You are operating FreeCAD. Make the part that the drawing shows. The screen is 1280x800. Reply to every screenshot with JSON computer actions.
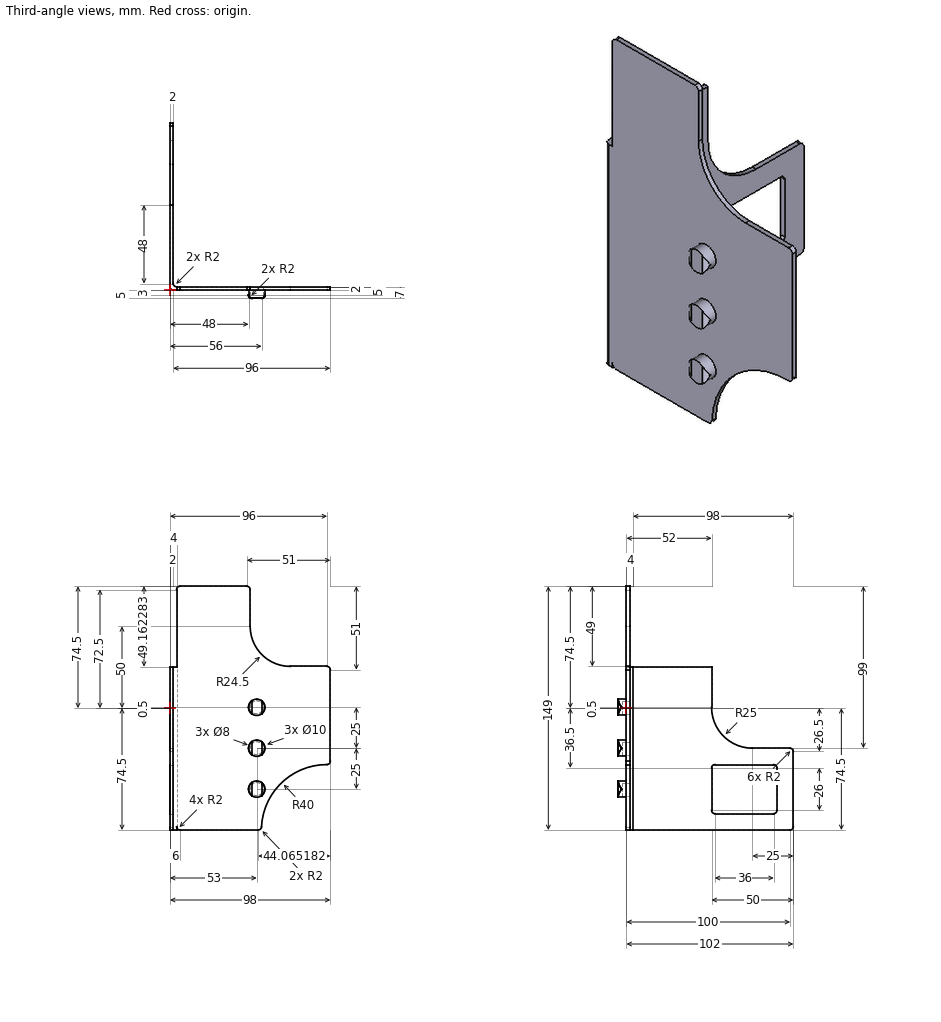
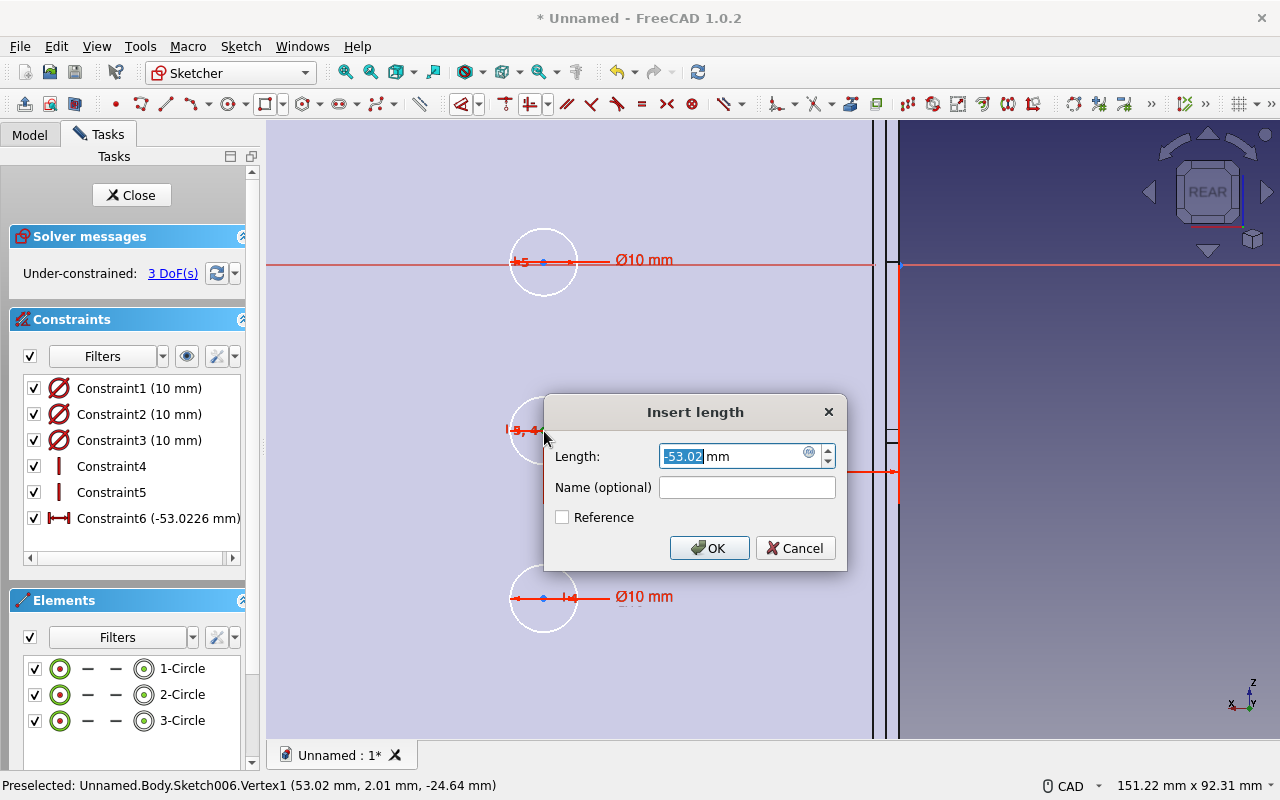
{"action": "type", "text": "-53"}
{"action": "key", "text": "Return"}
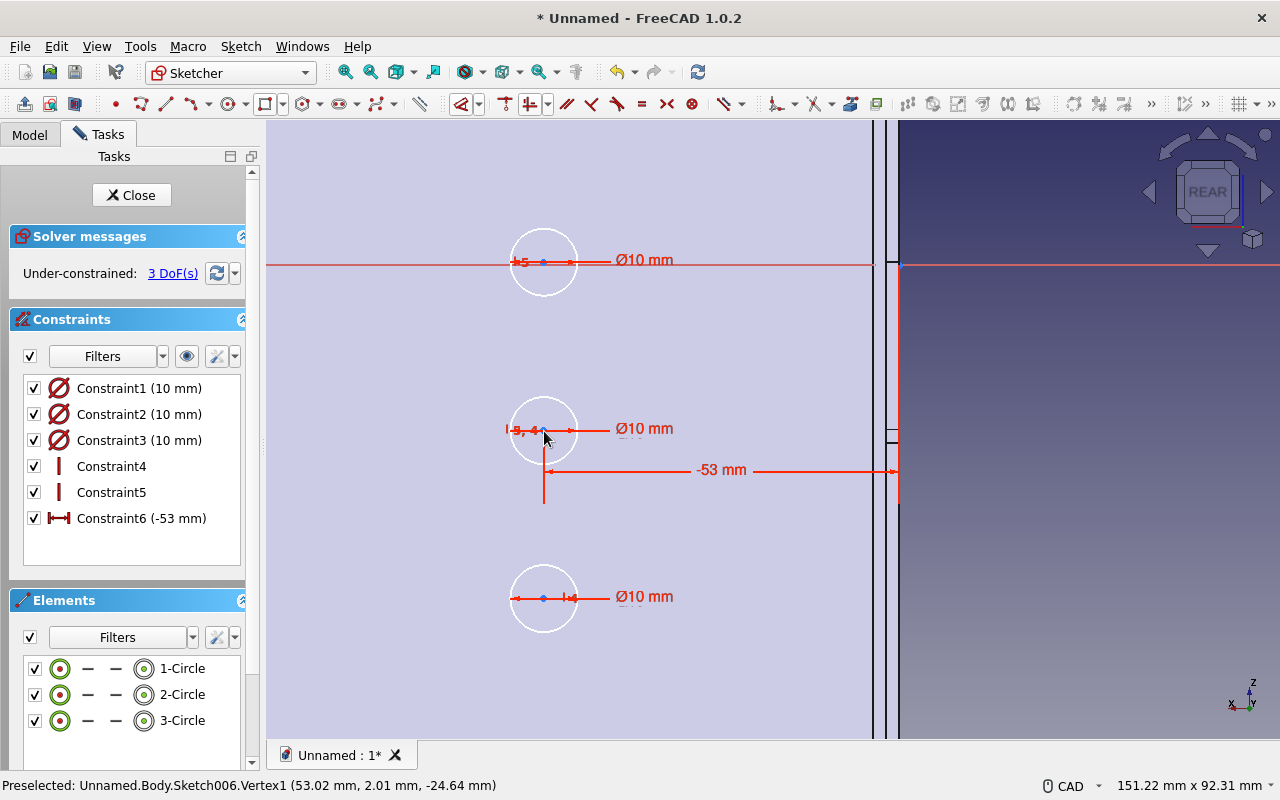
{"action": "scroll", "coordinate": [544, 262], "scroll_direction": "up", "scroll_amount": 13}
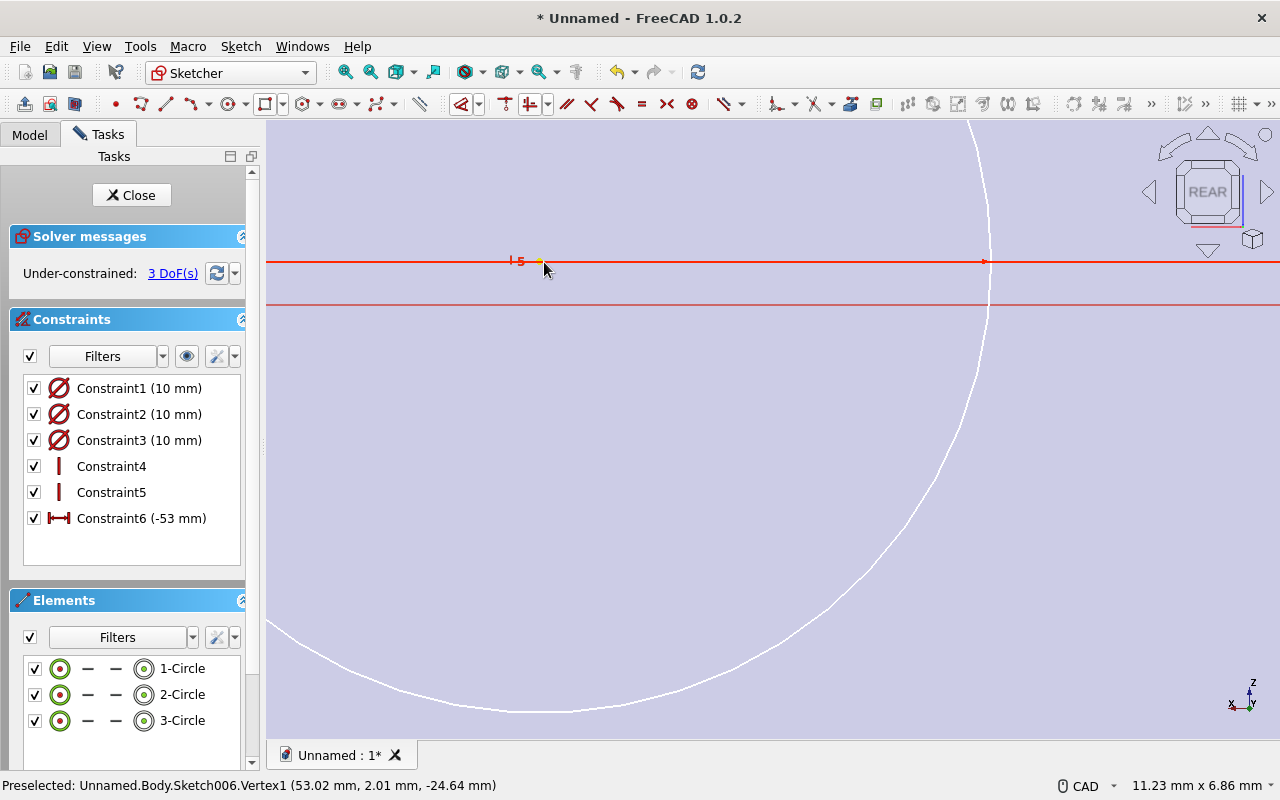
{"action": "left_click", "coordinate": [540, 262]}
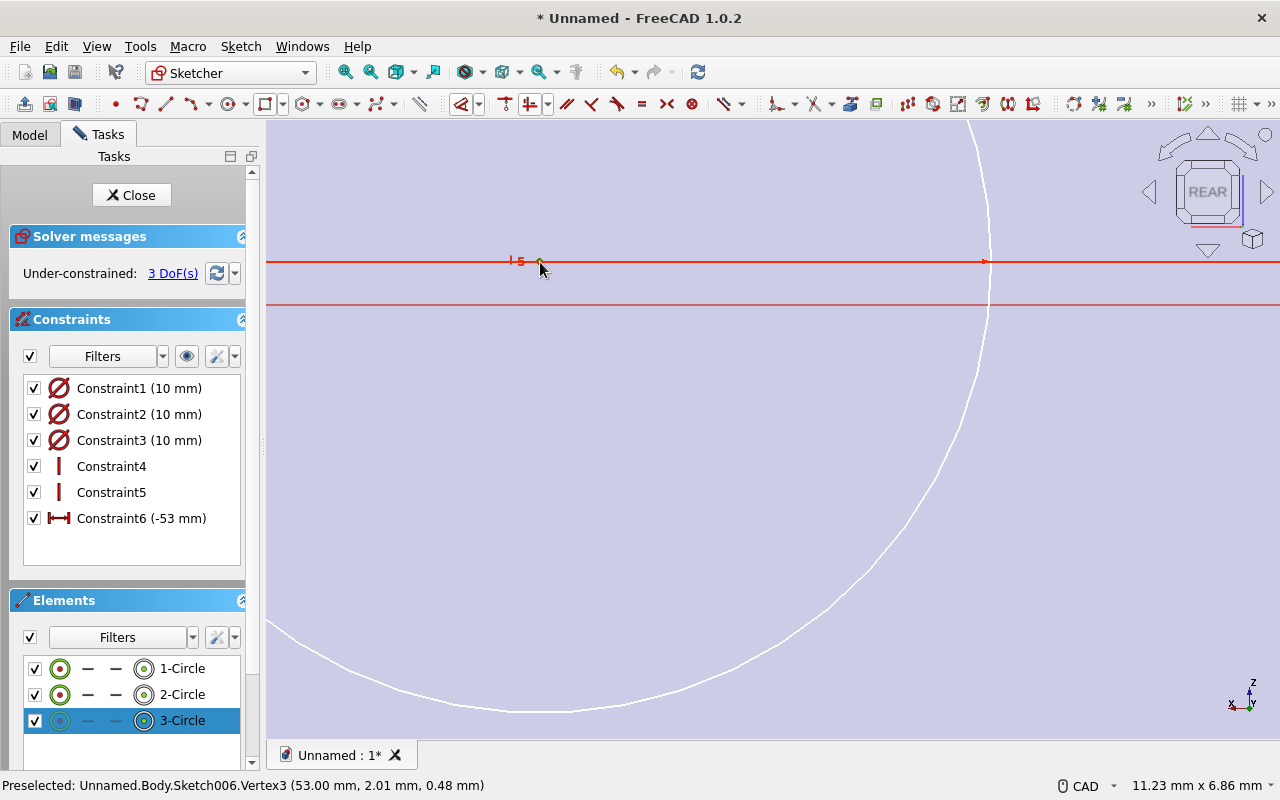
{"action": "key", "text": "i"}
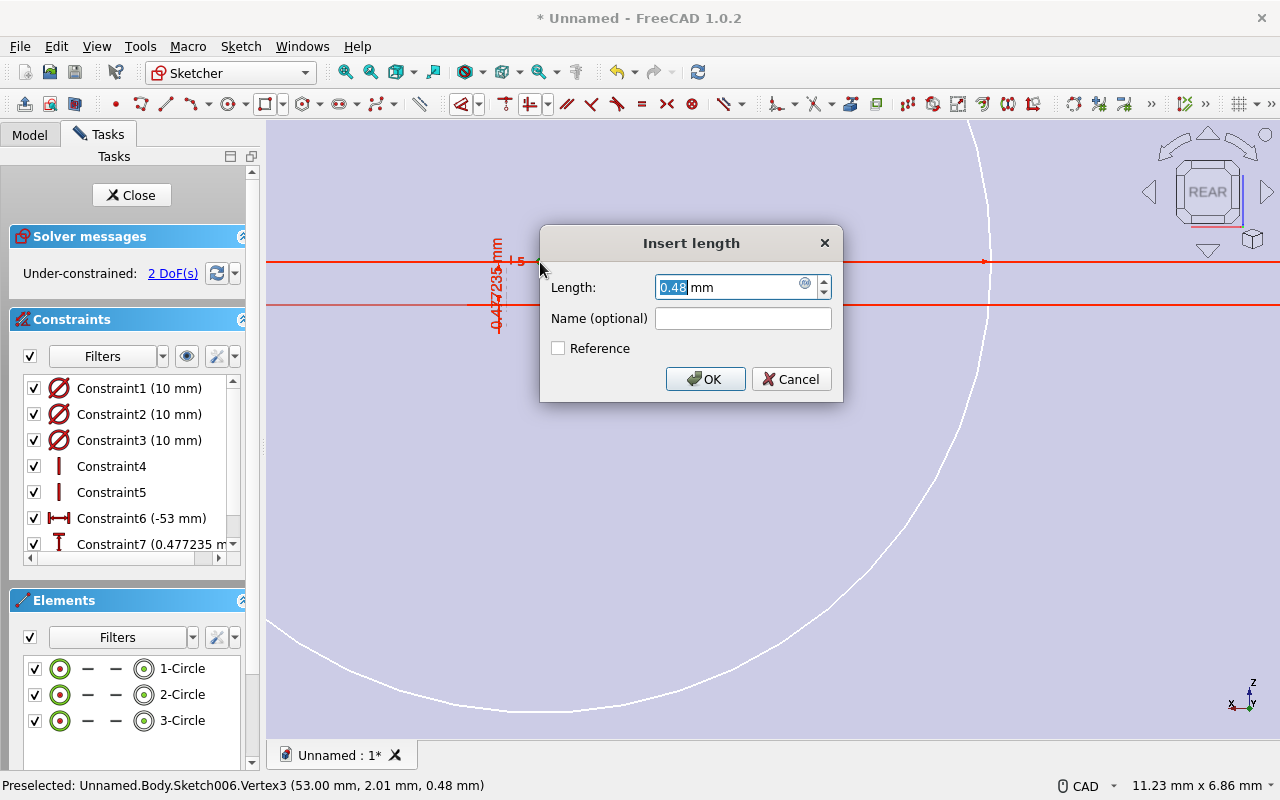
{"action": "type", "text": "0.5"}
{"action": "key", "text": "Return"}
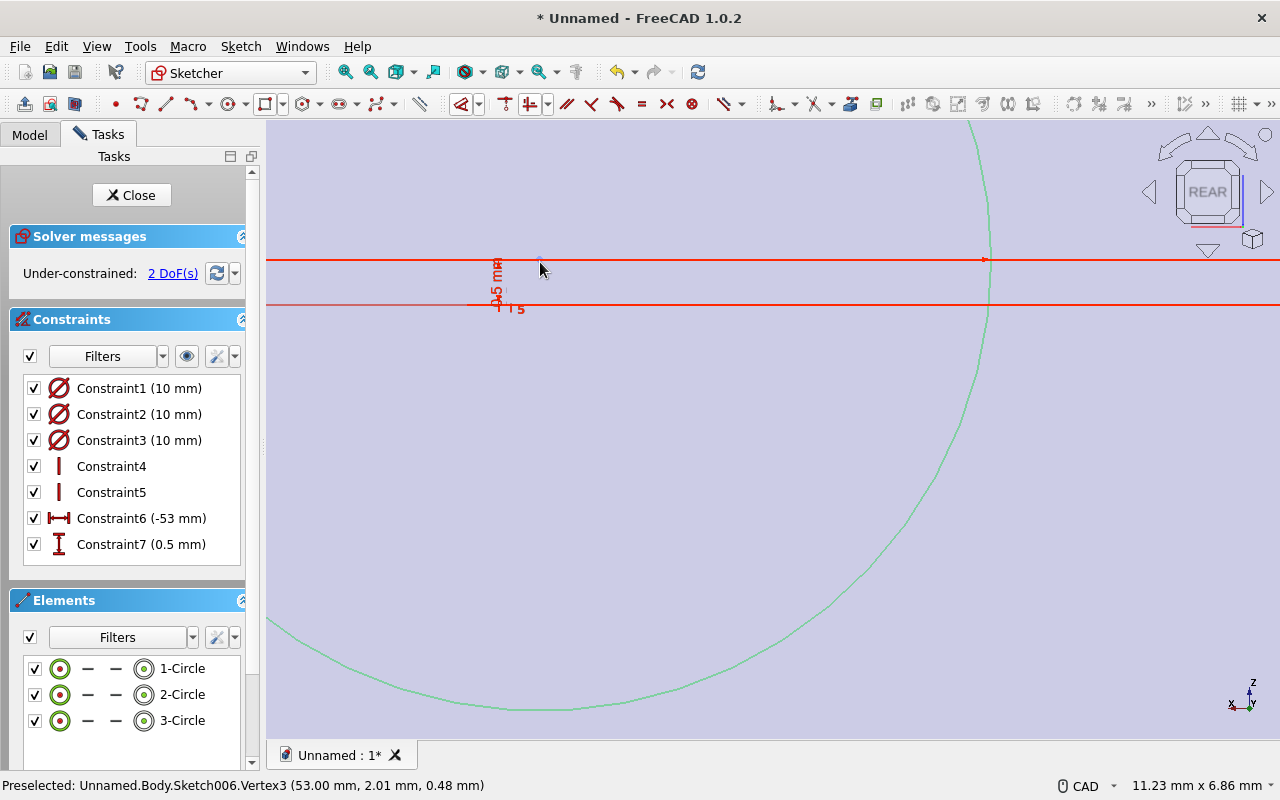
{"action": "scroll", "coordinate": [544, 262], "scroll_direction": "down", "scroll_amount": 13}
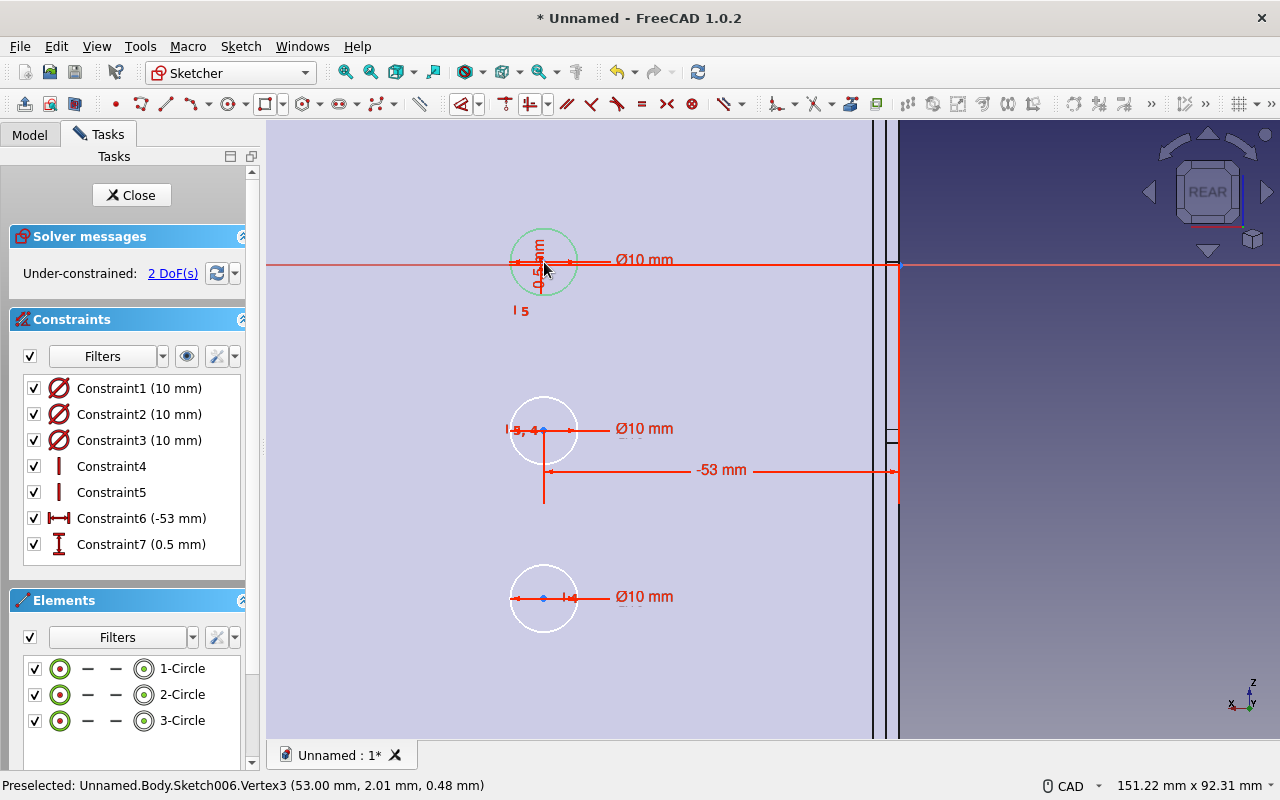
{"action": "left_click", "coordinate": [544, 431]}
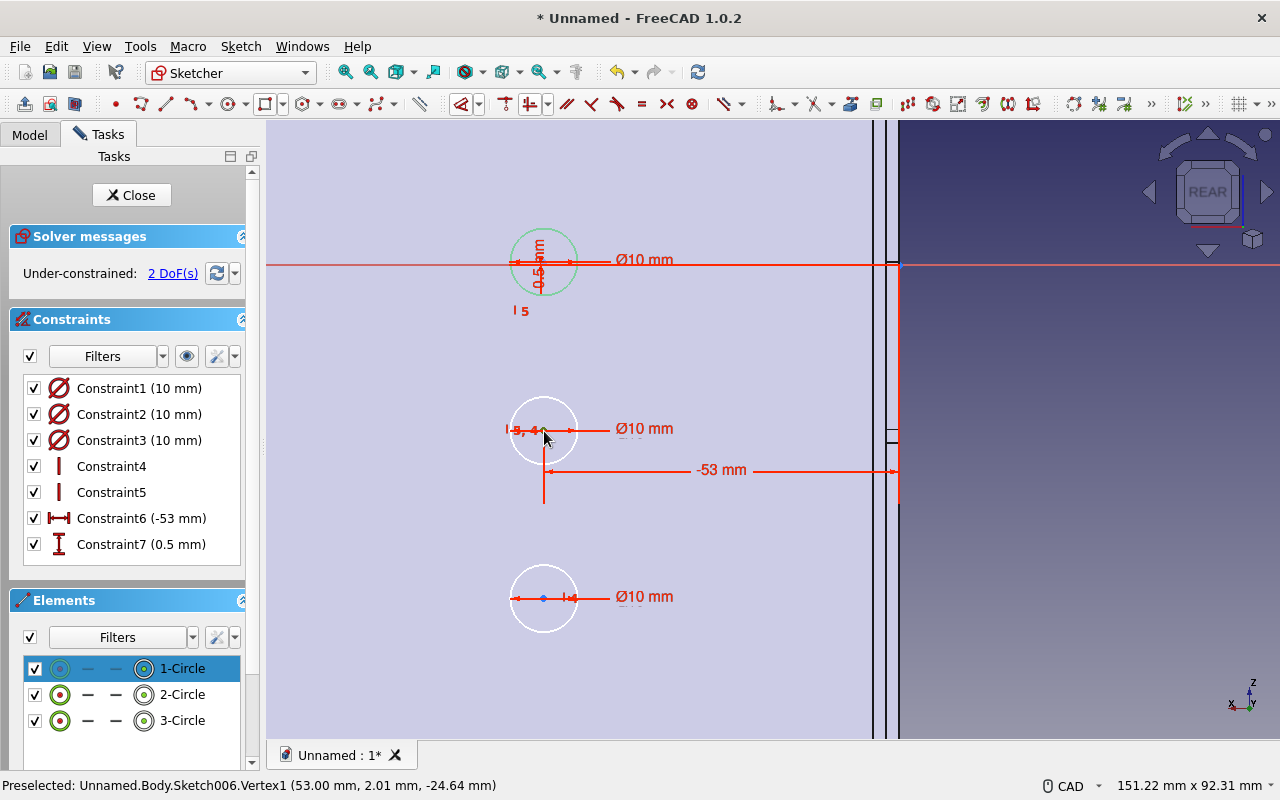
{"action": "left_click", "coordinate": [544, 599]}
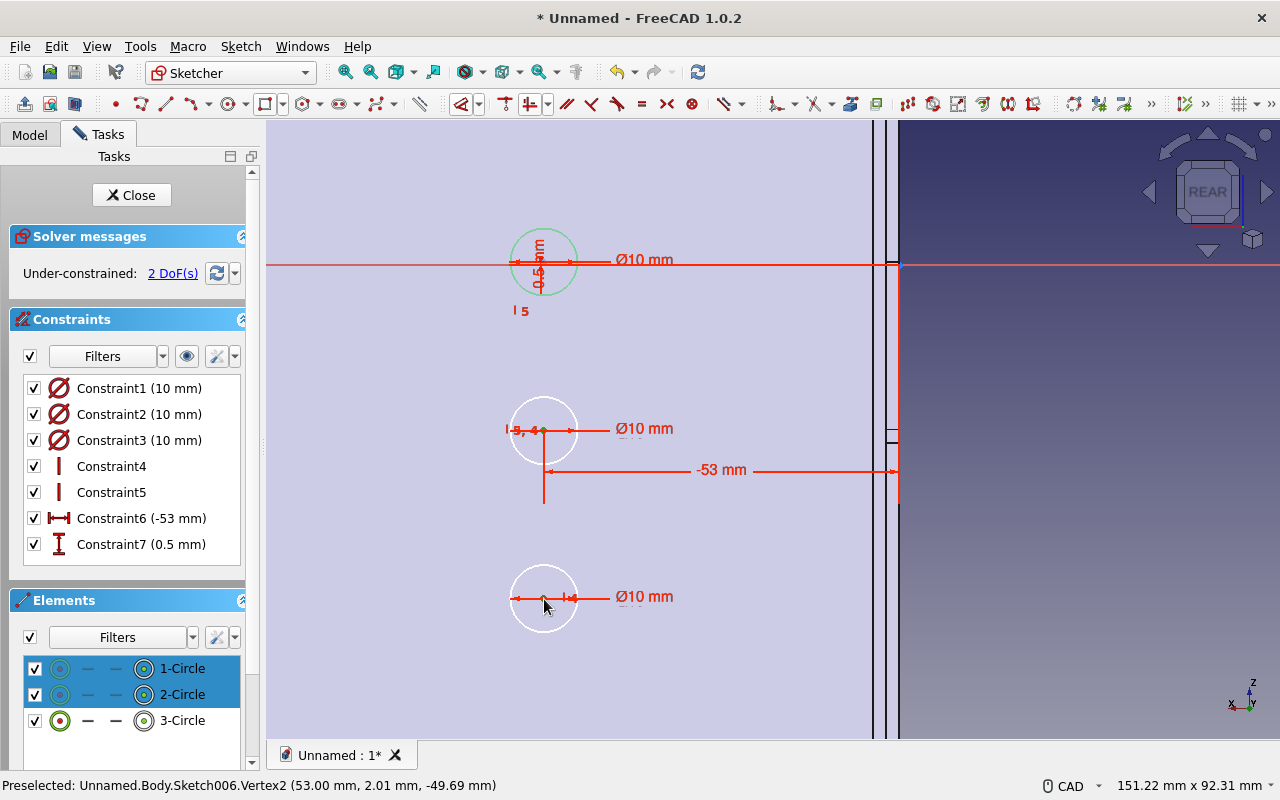
{"action": "left_click", "coordinate": [478, 104]}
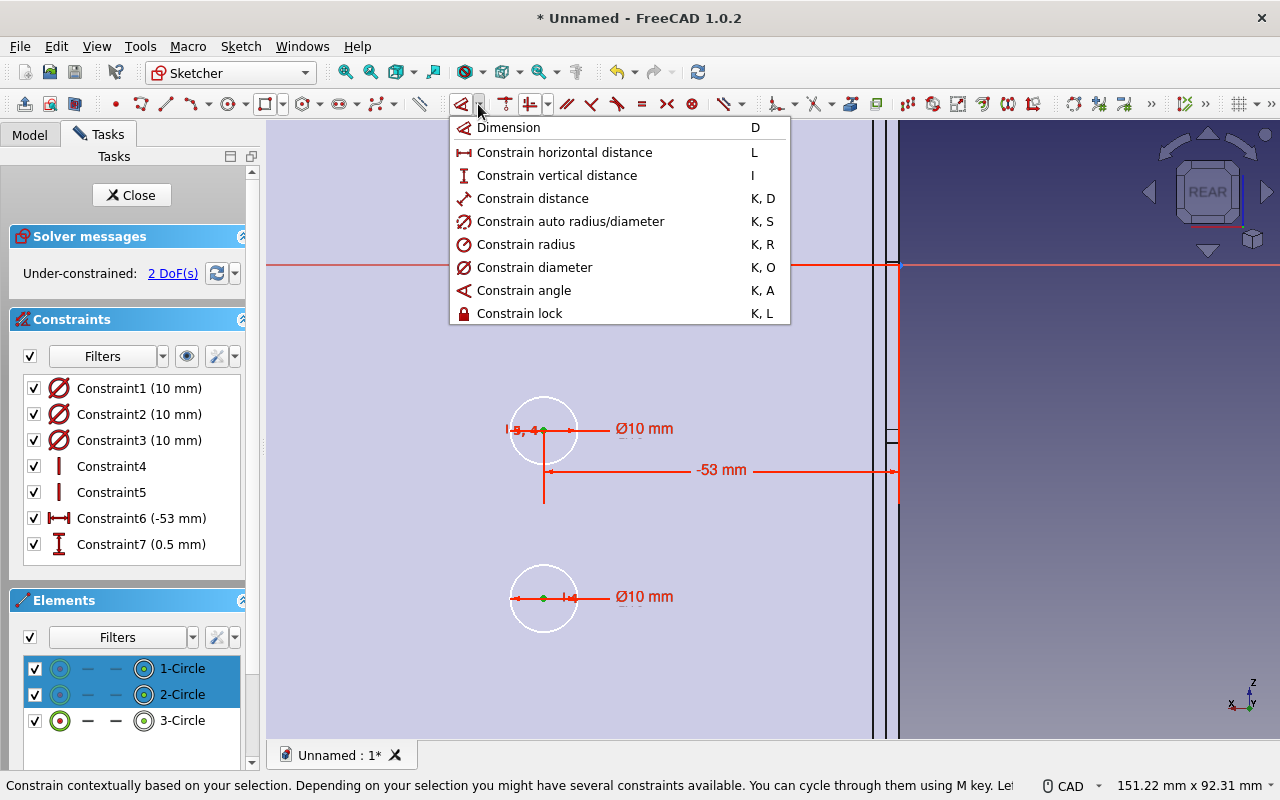
{"action": "left_click", "coordinate": [620, 176]}